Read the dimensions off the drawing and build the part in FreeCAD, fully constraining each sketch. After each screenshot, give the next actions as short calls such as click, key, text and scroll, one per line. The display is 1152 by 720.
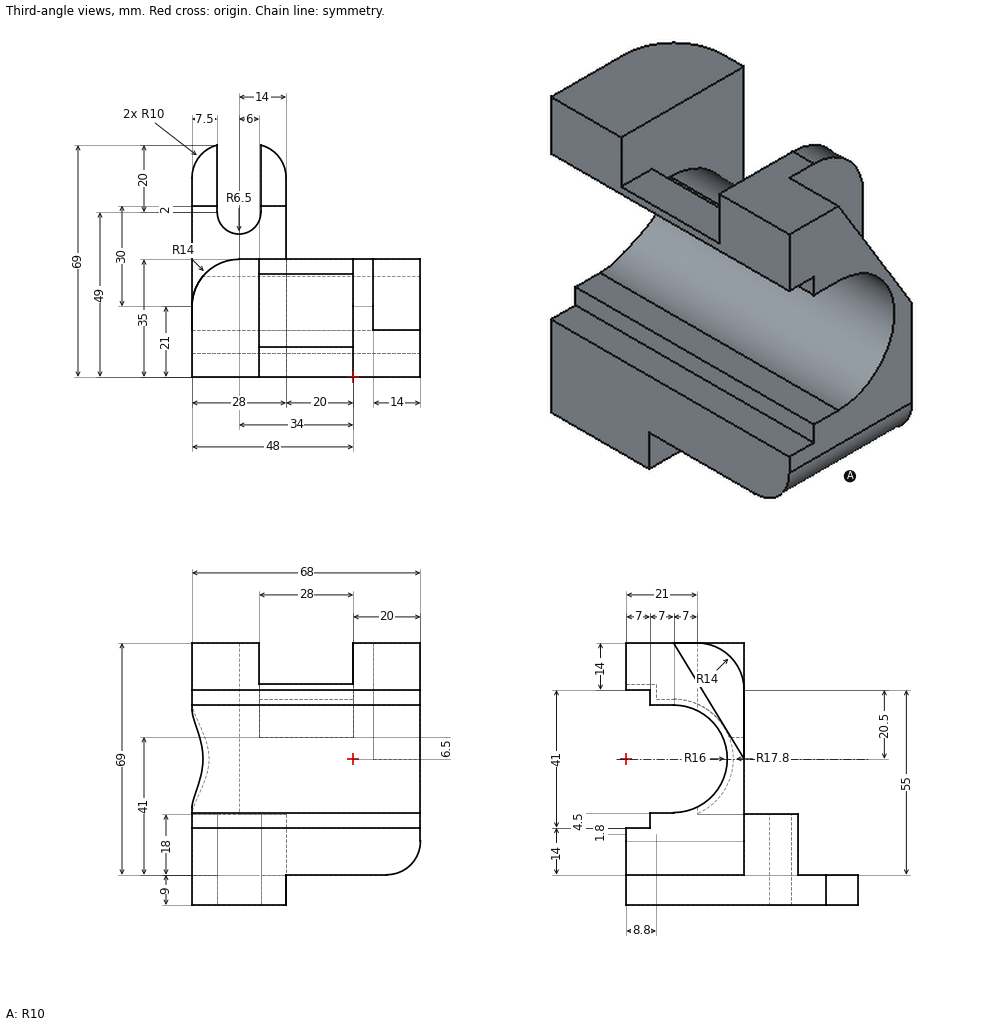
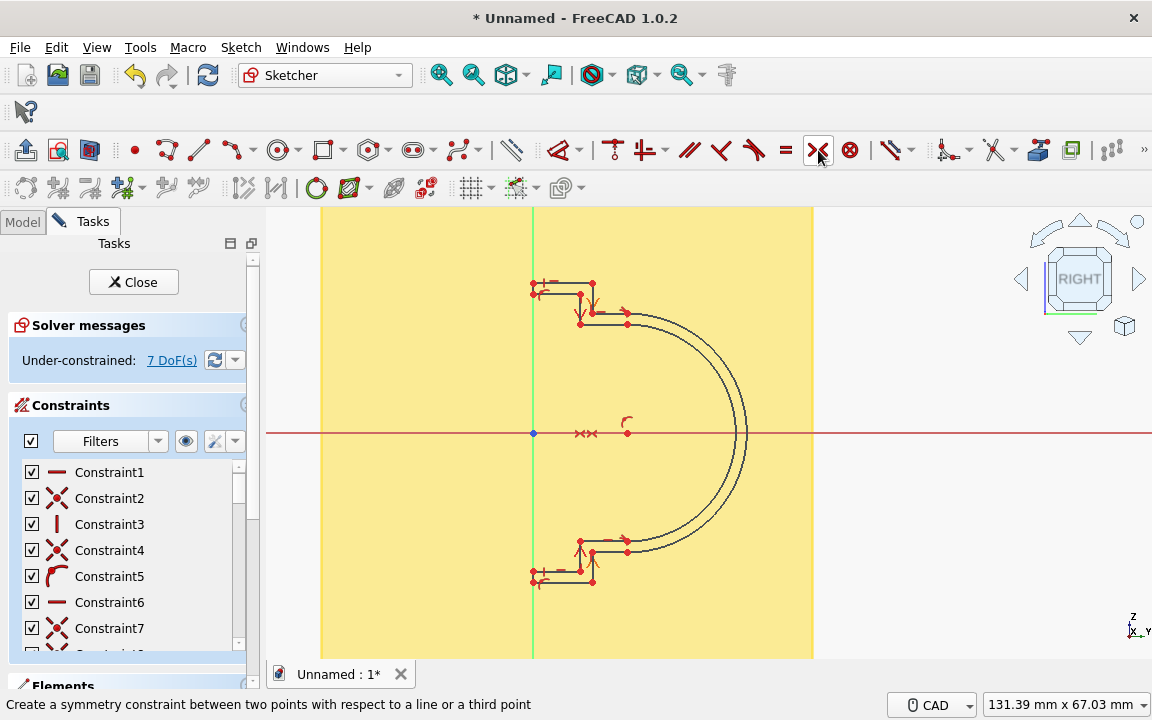
click(558, 150)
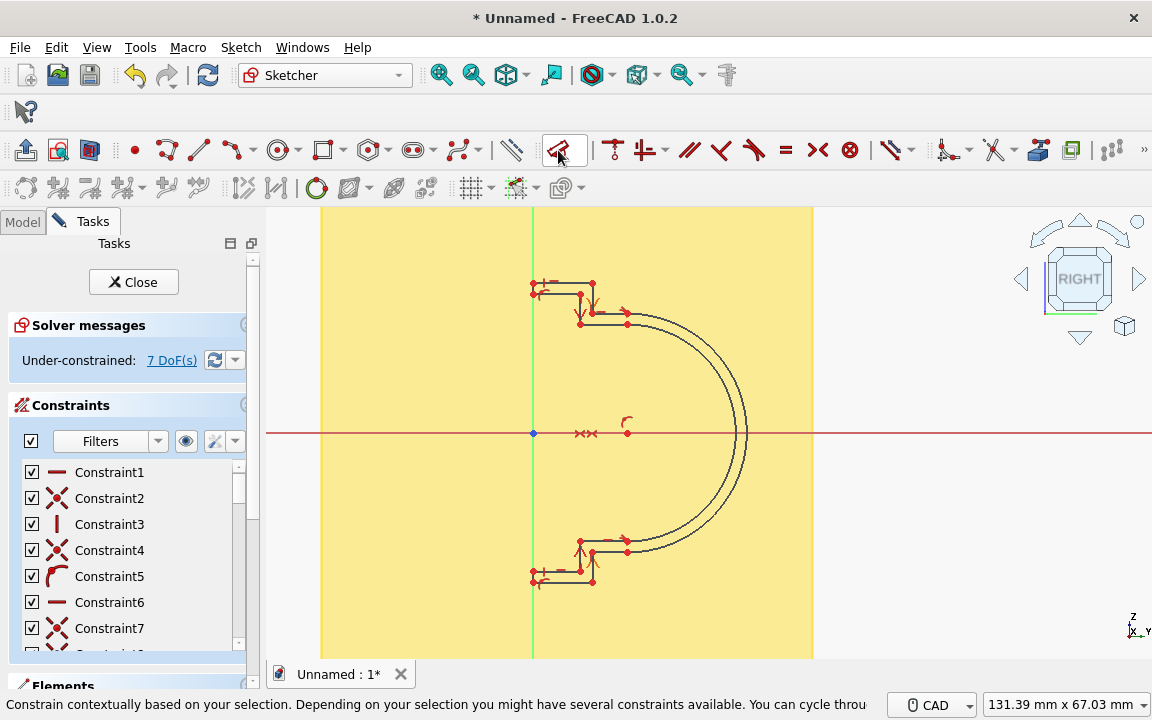
scroll(724, 503, up, 2)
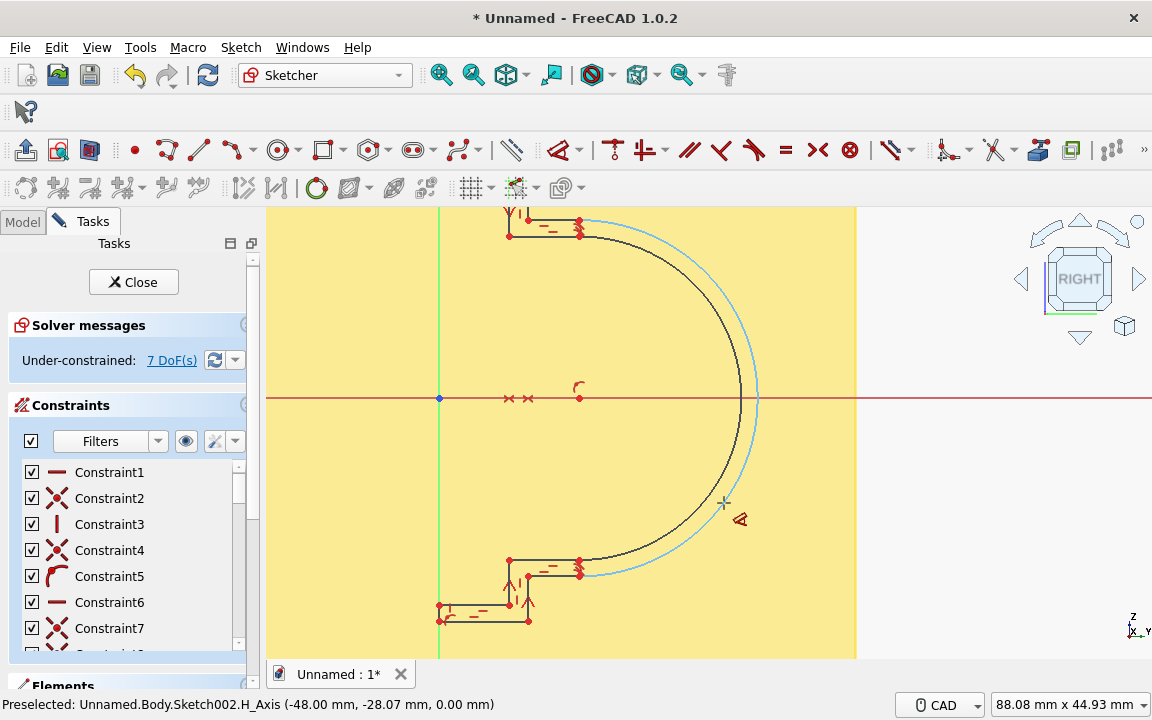
click(724, 503)
click(750, 522)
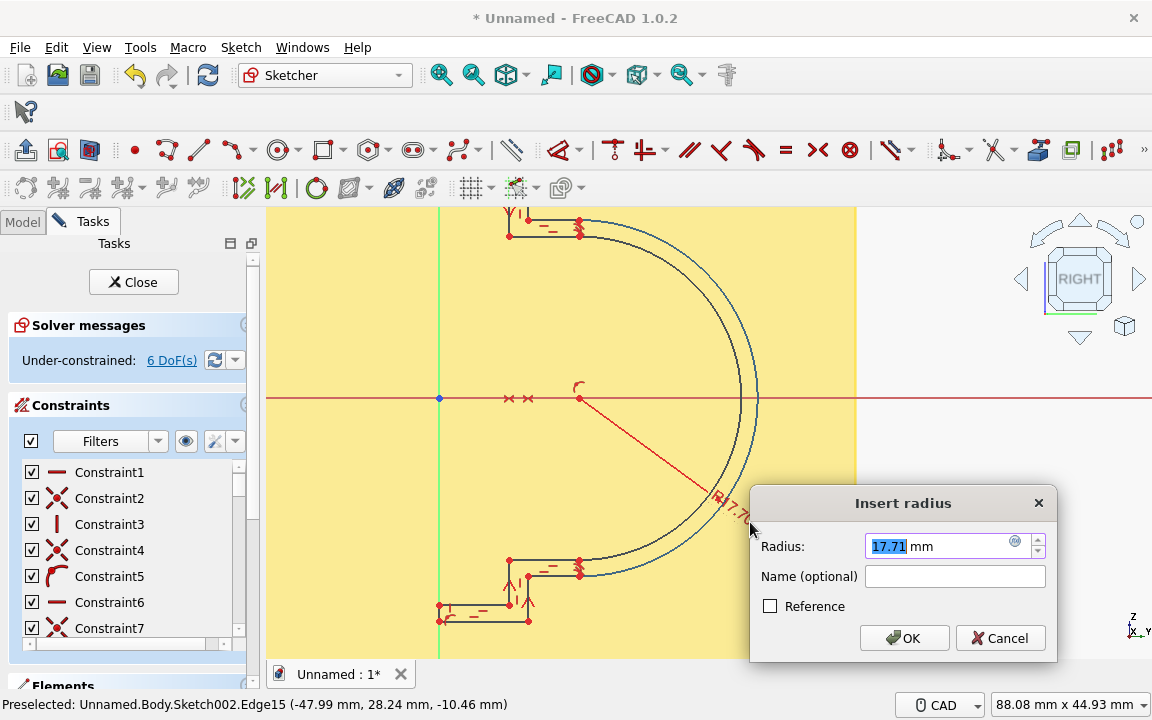
text(17.8)
key(Return)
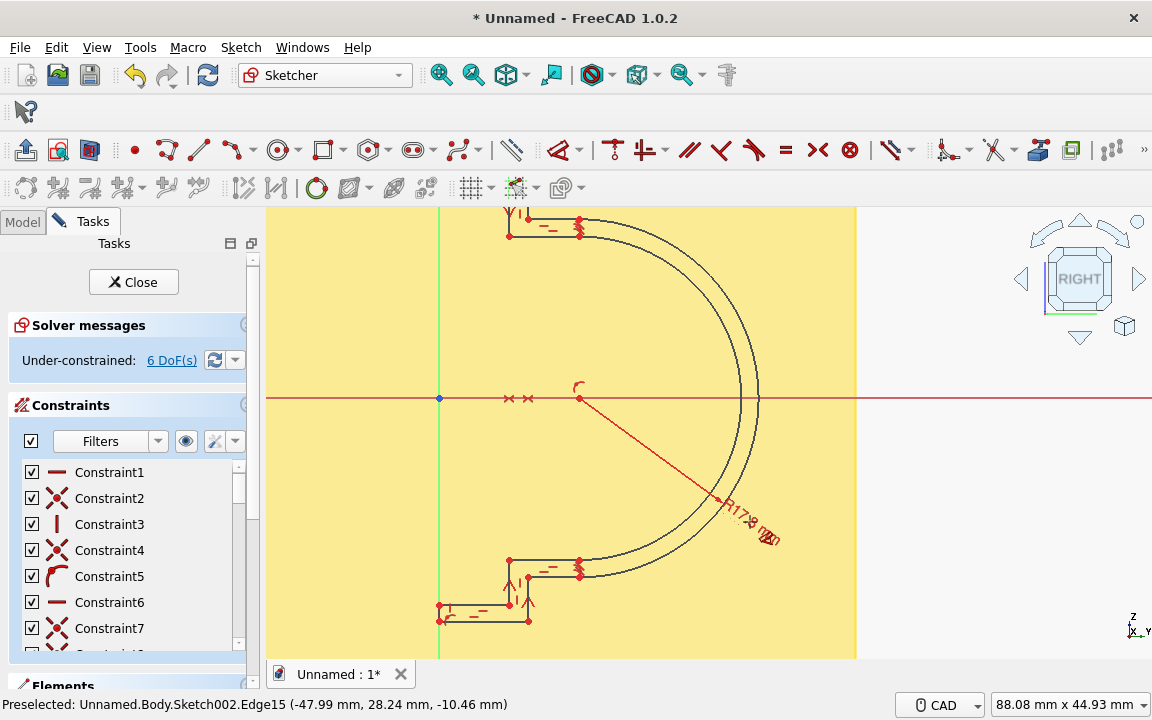
click(710, 493)
click(662, 573)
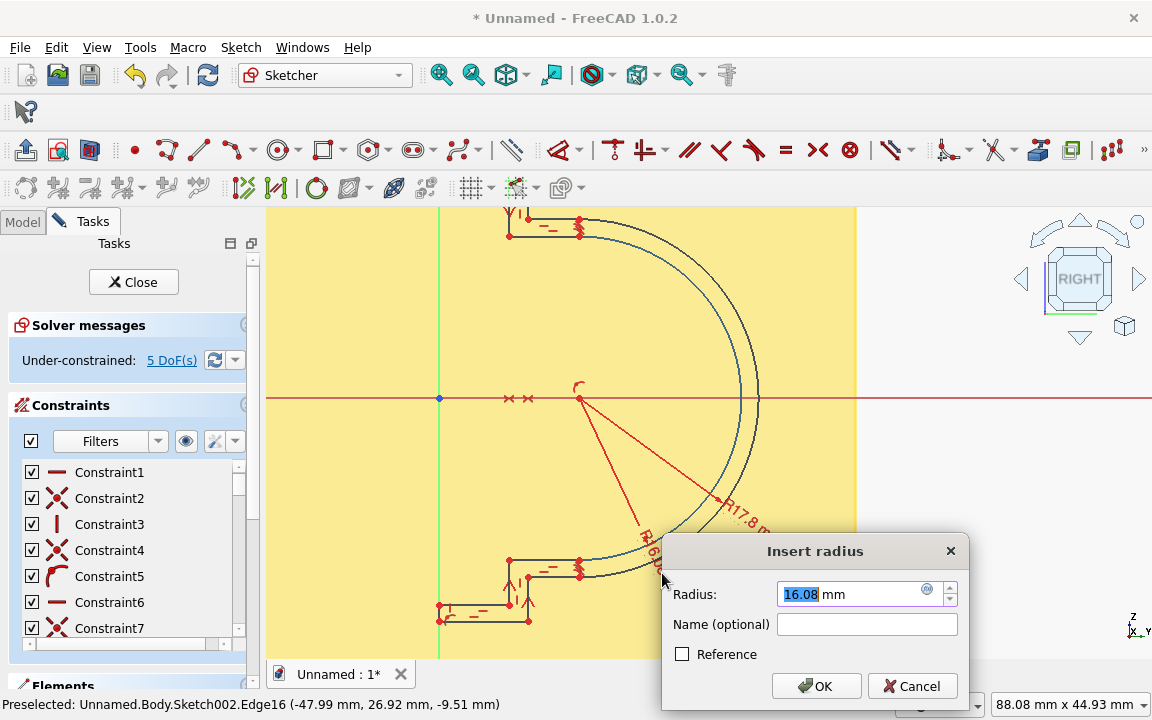
text(16)
key(Return)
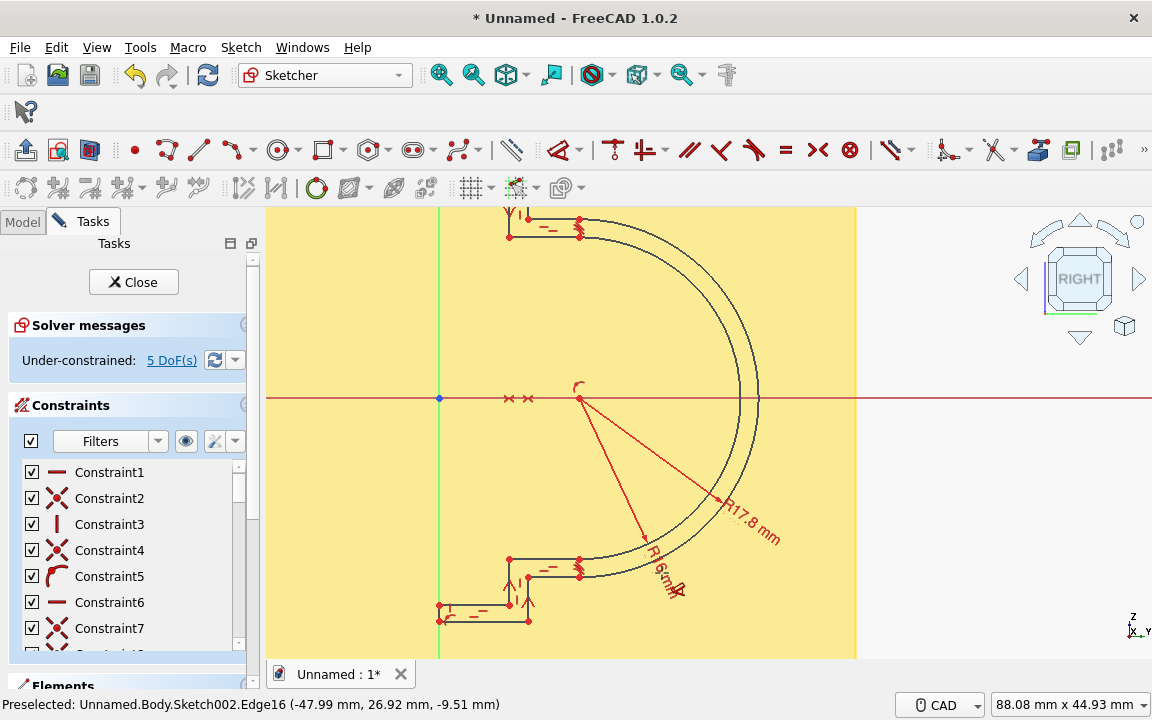
click(559, 559)
click(545, 593)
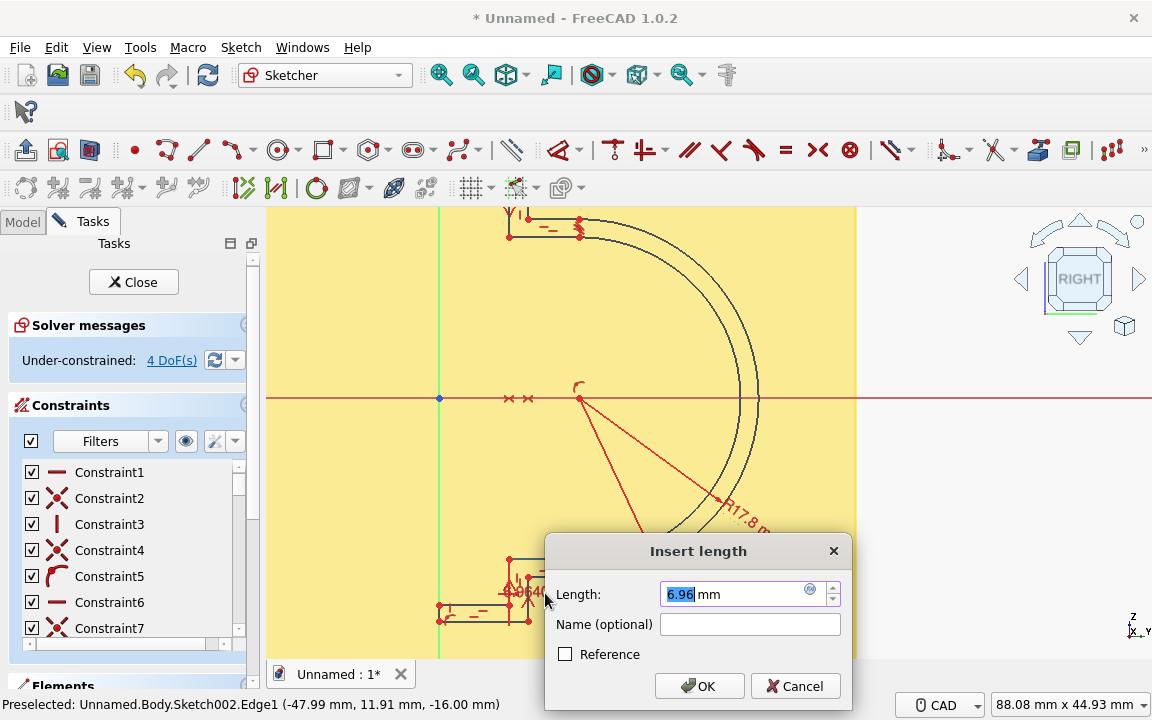
text(7)
key(Return)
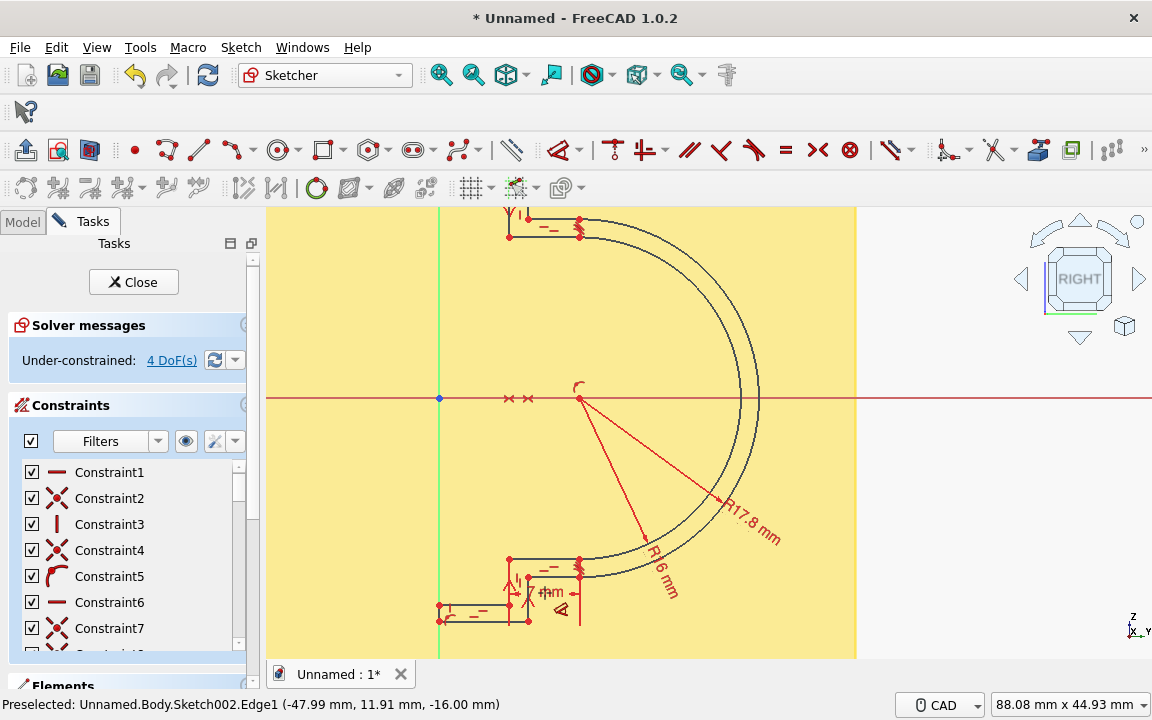
click(488, 605)
click(474, 571)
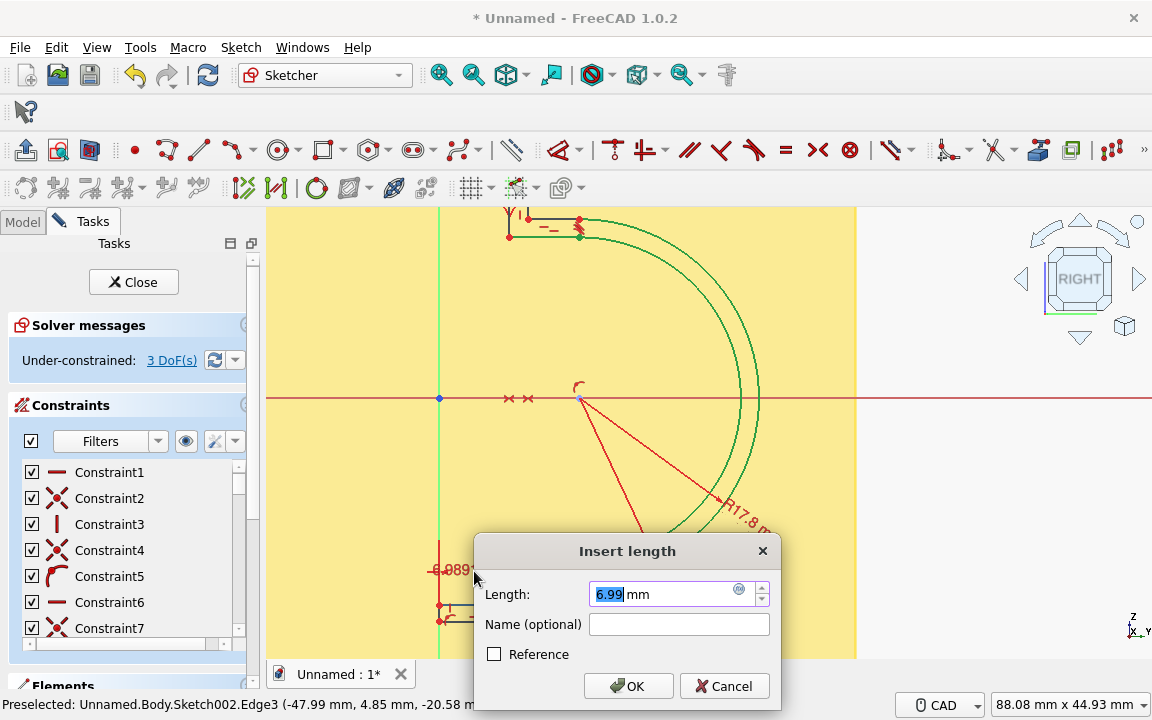
text(7)
key(Return)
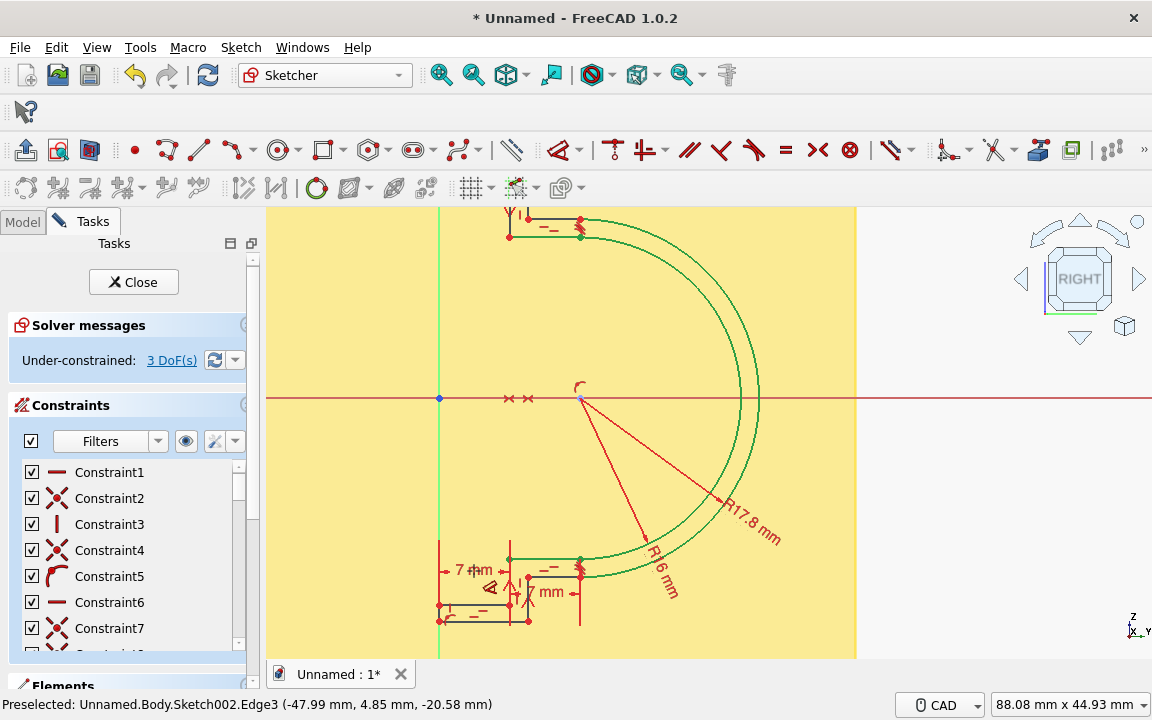
click(510, 573)
click(404, 582)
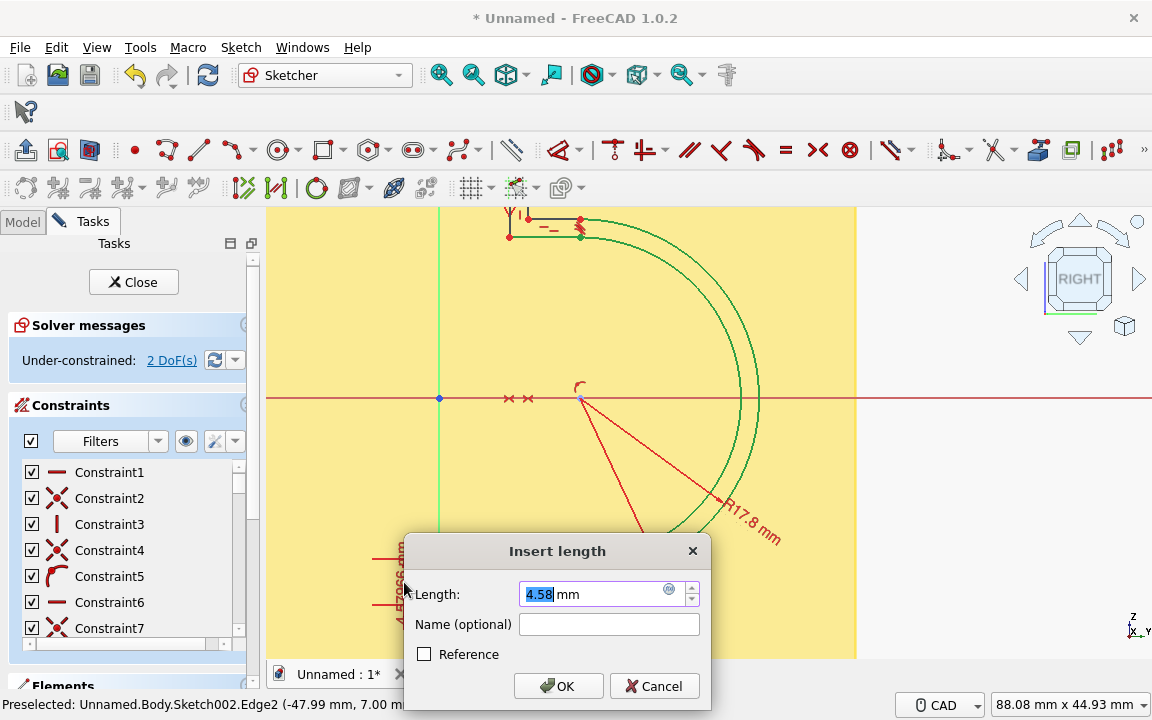
text(4.5)
key(Return)